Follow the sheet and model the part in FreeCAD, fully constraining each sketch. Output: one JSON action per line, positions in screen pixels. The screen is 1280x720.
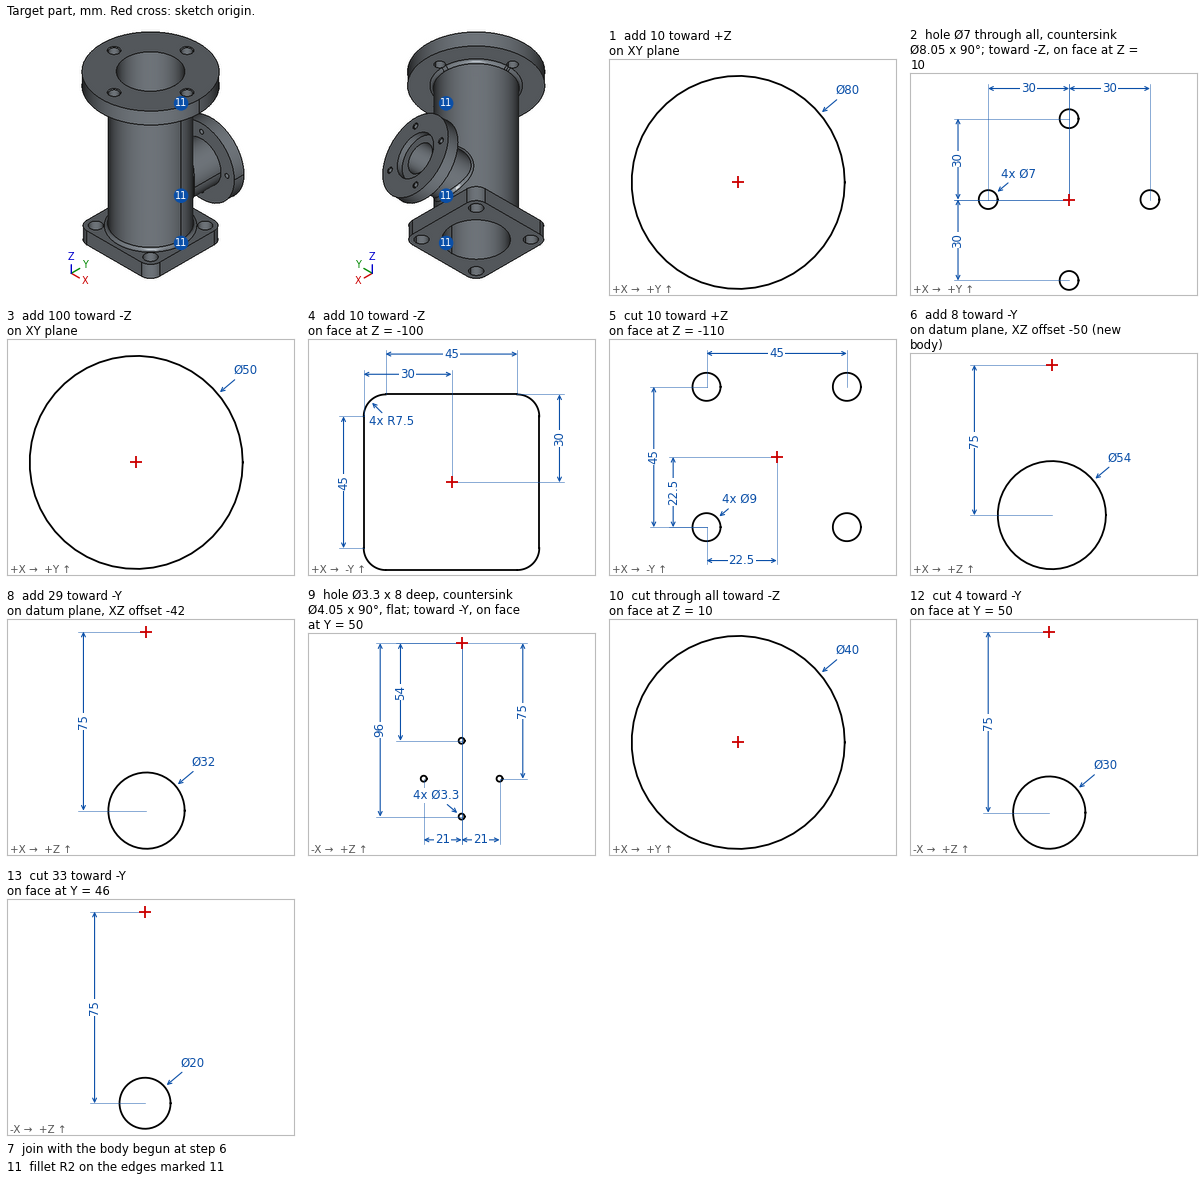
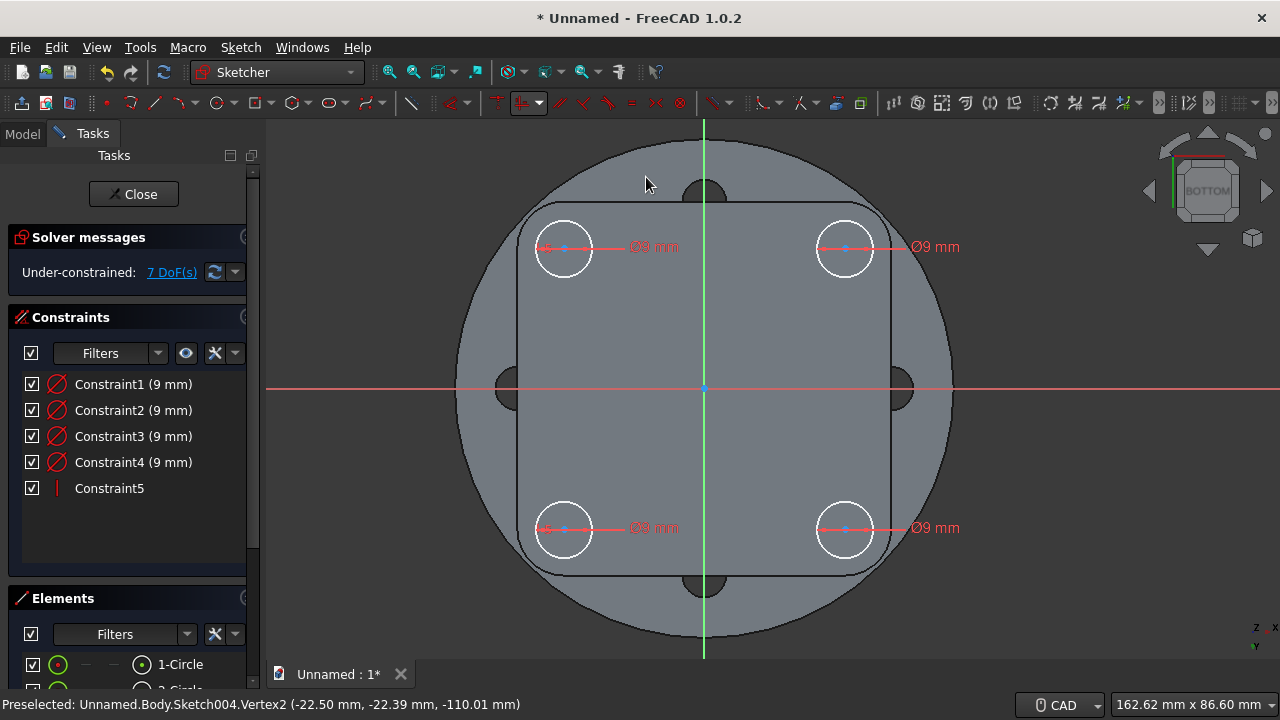
{"action": "left_click", "coordinate": [564, 249]}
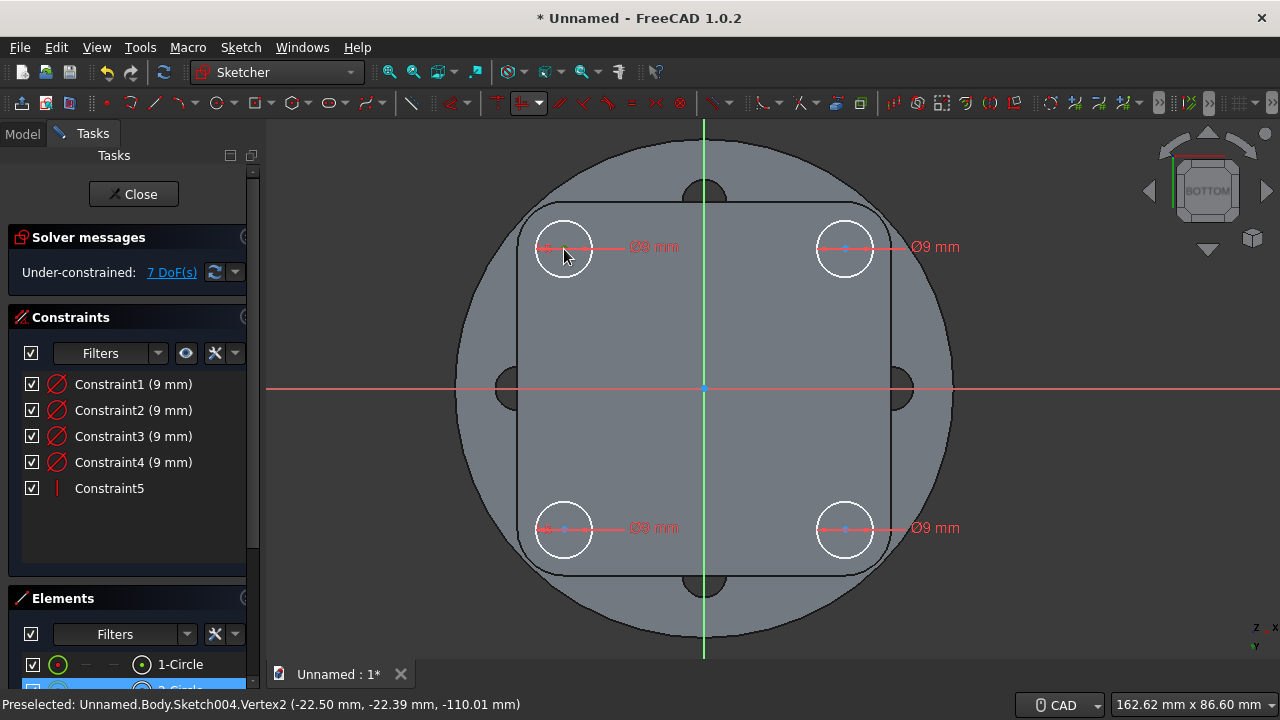
{"action": "left_click", "coordinate": [845, 249]}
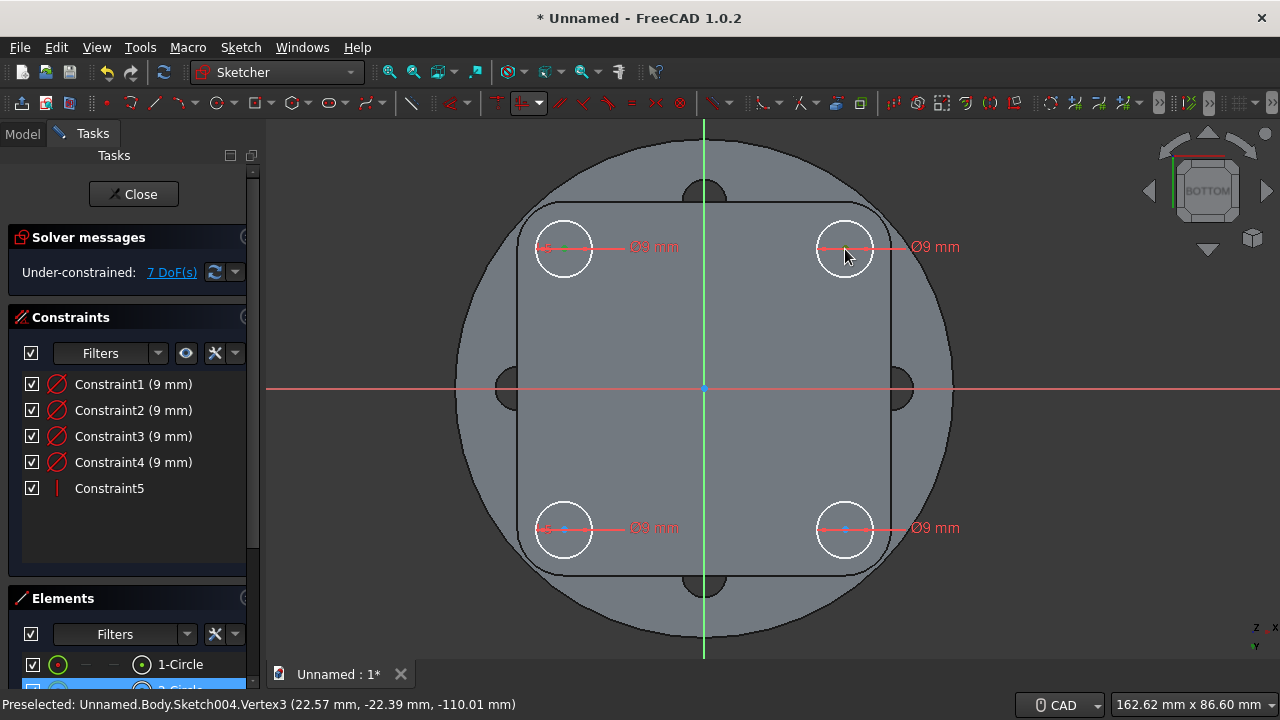
{"action": "left_click", "coordinate": [542, 104]}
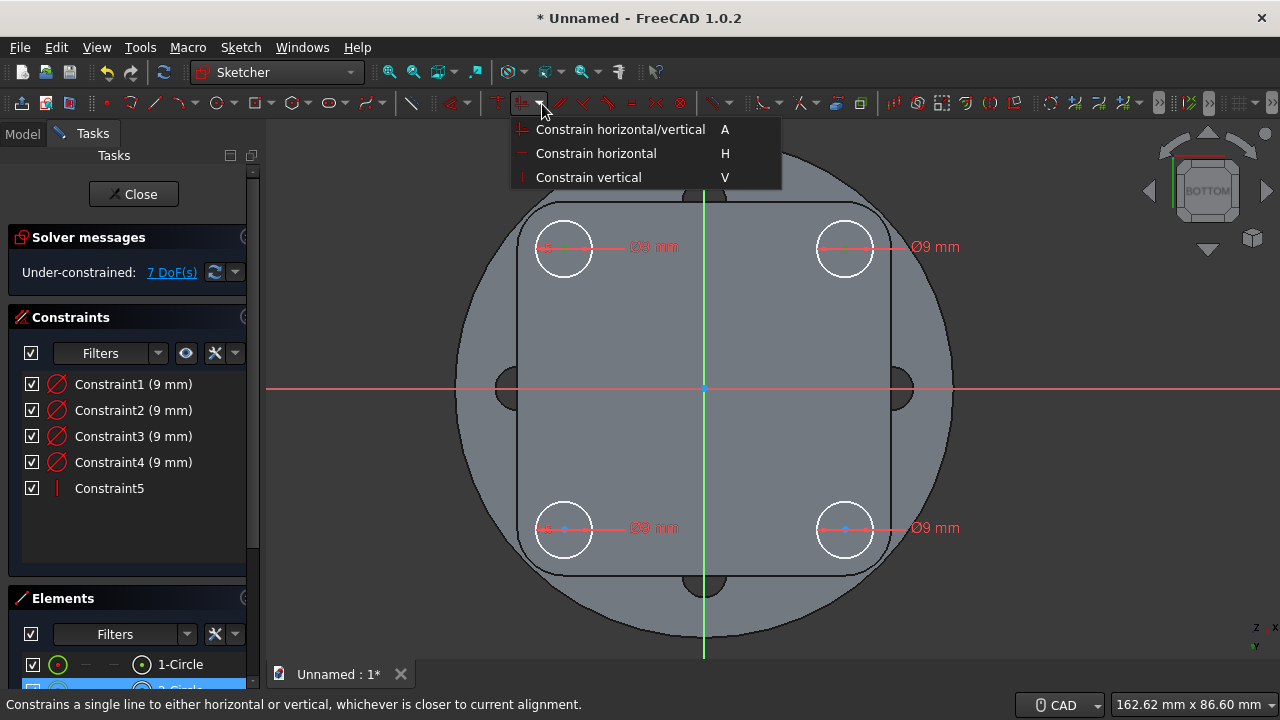
{"action": "left_click", "coordinate": [646, 153]}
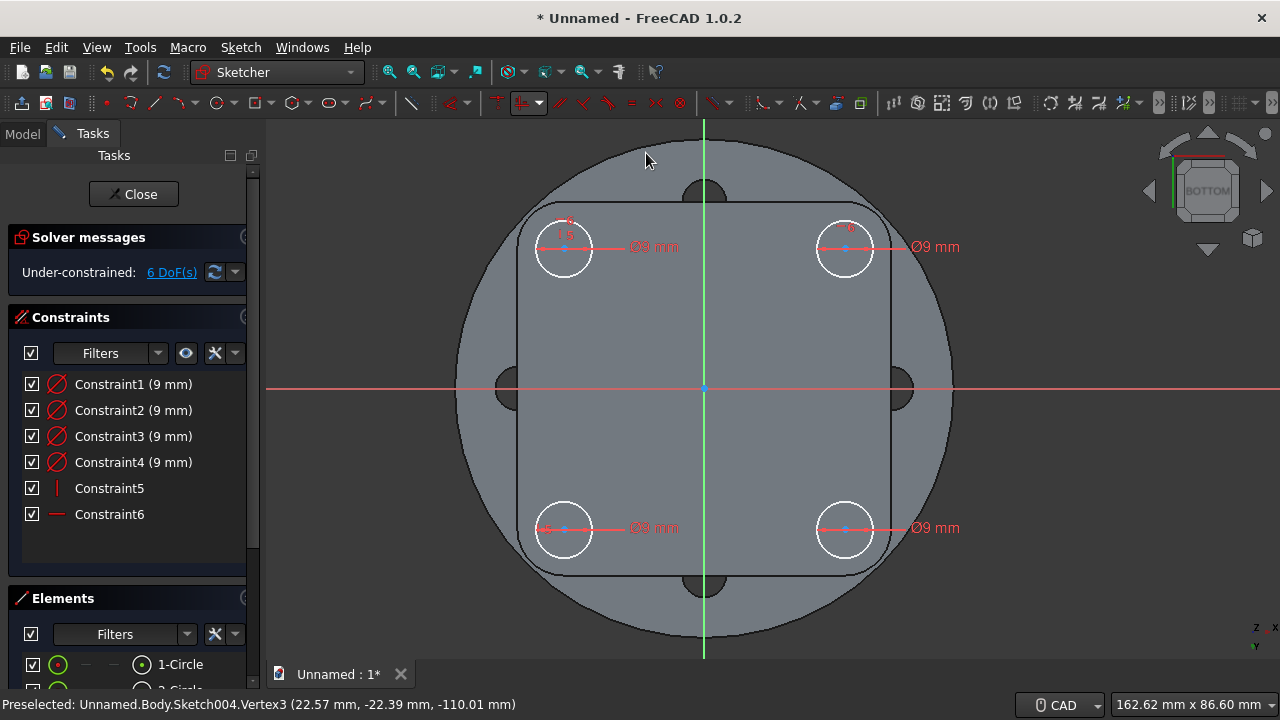
{"action": "left_click", "coordinate": [845, 249]}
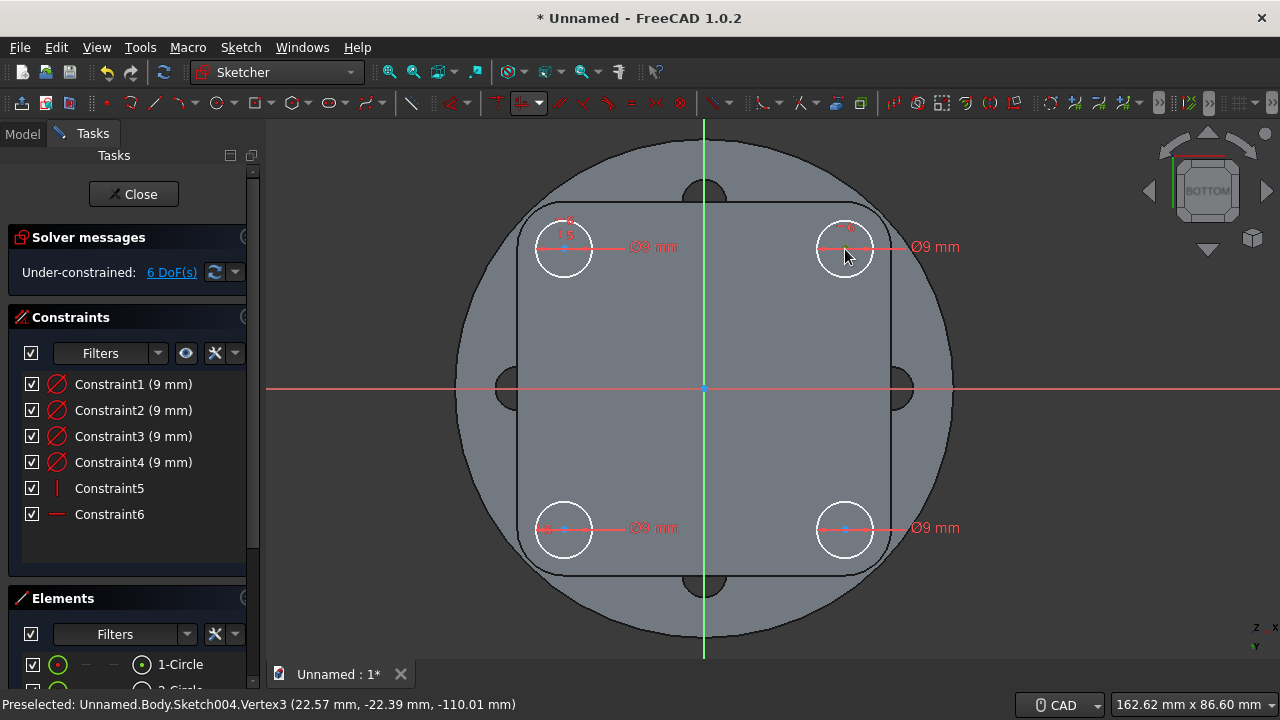
{"action": "left_click", "coordinate": [845, 530]}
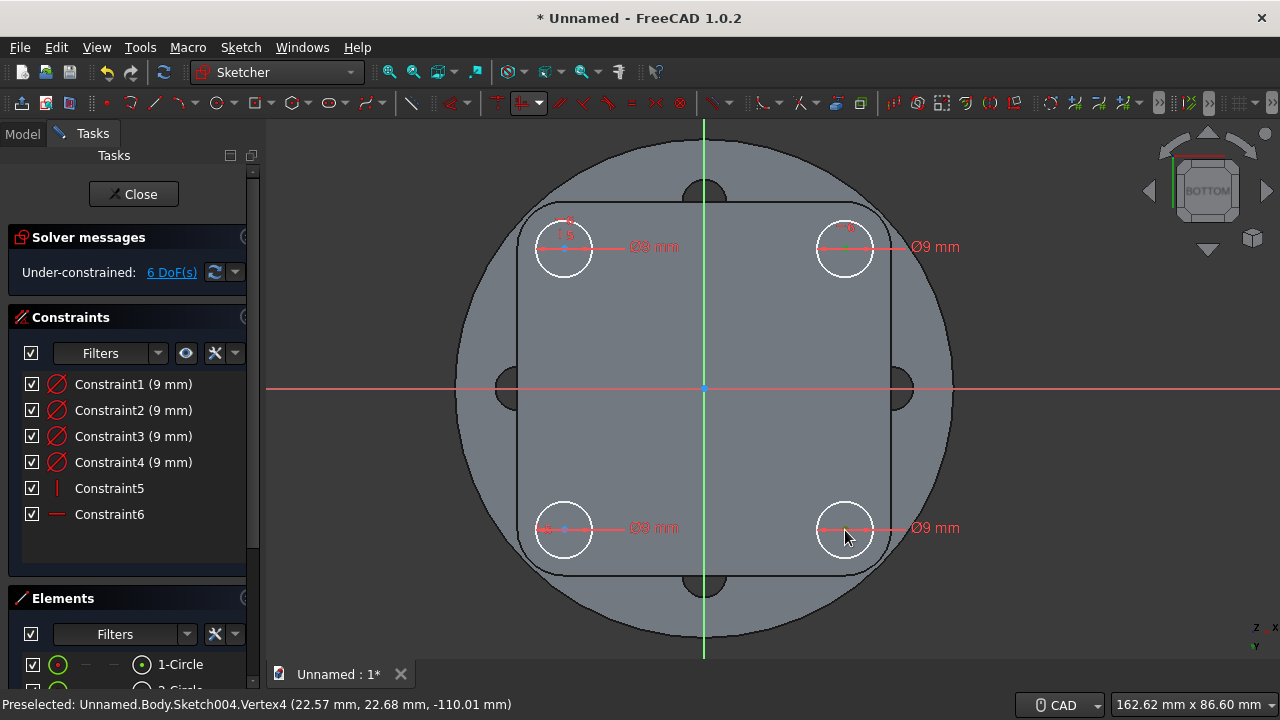
{"action": "left_click", "coordinate": [542, 104]}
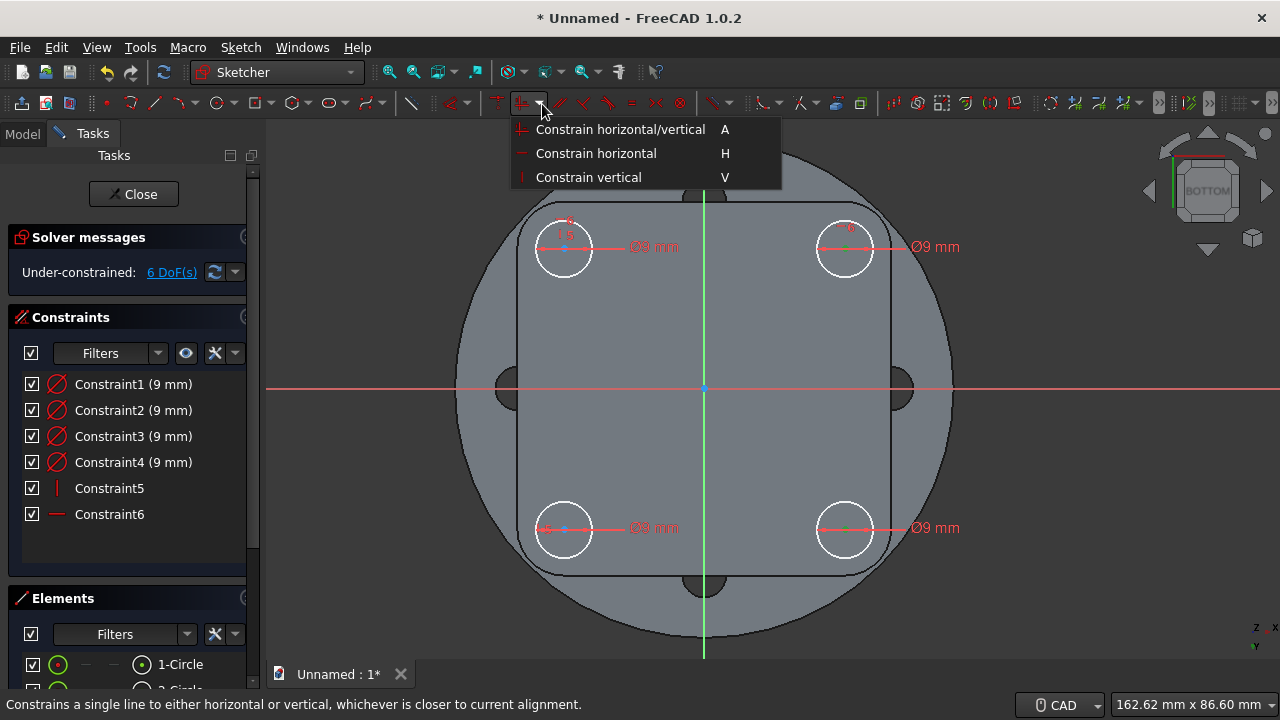
{"action": "left_click", "coordinate": [646, 177]}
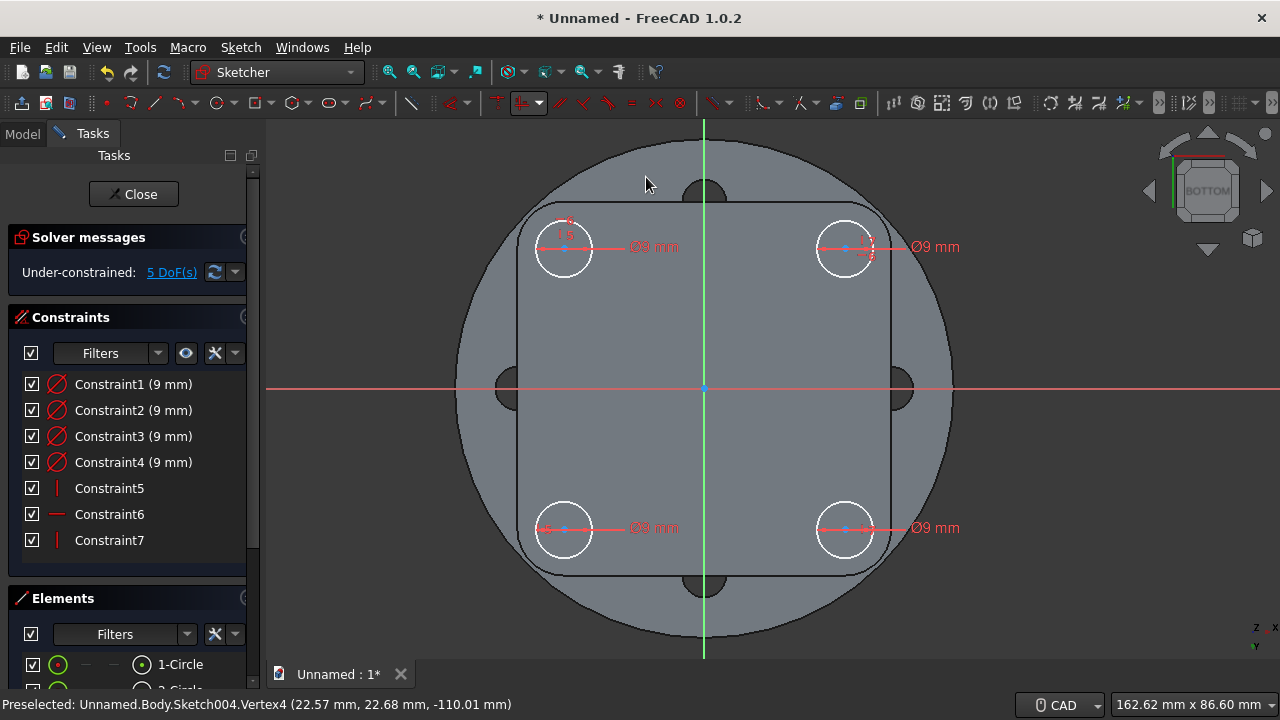
{"action": "left_click", "coordinate": [564, 530]}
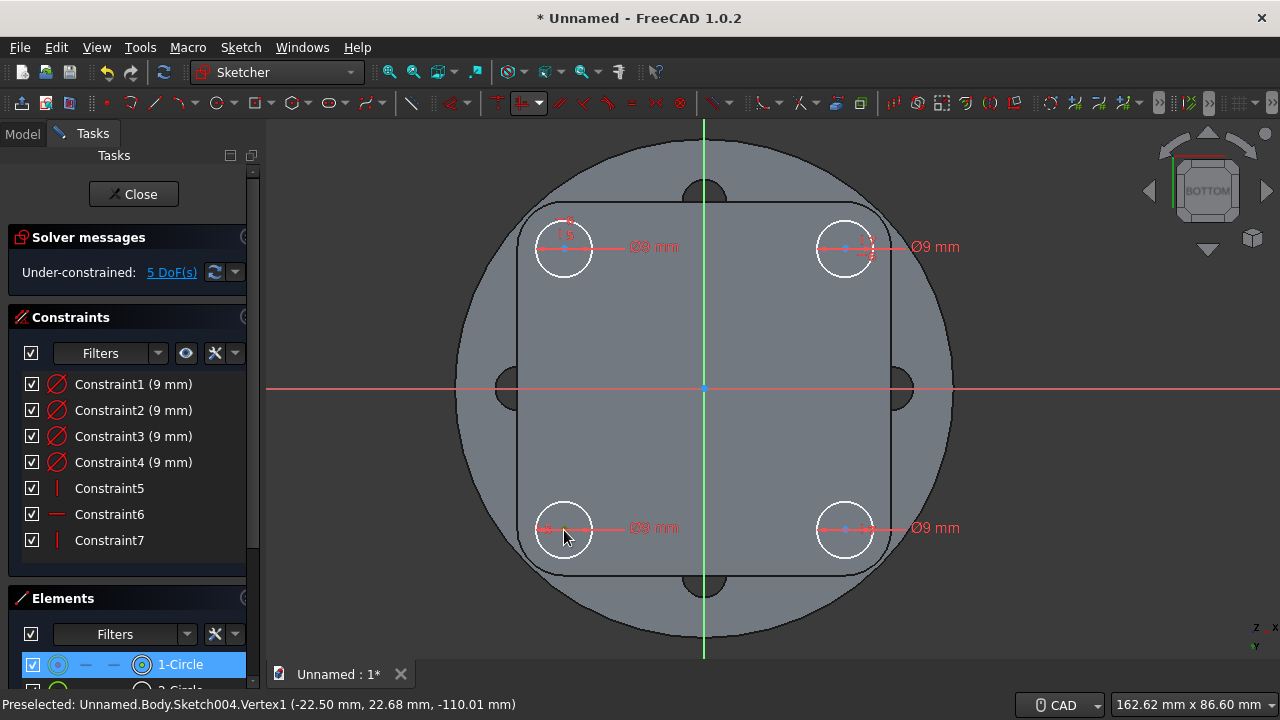
{"action": "left_click", "coordinate": [845, 530]}